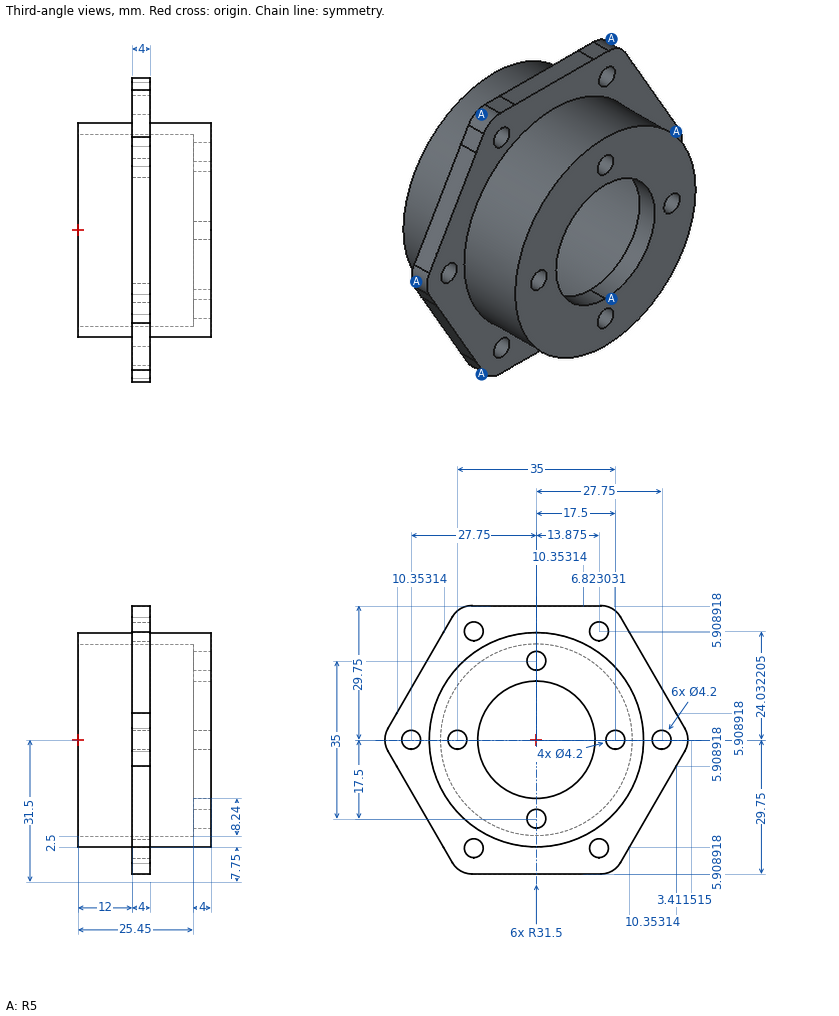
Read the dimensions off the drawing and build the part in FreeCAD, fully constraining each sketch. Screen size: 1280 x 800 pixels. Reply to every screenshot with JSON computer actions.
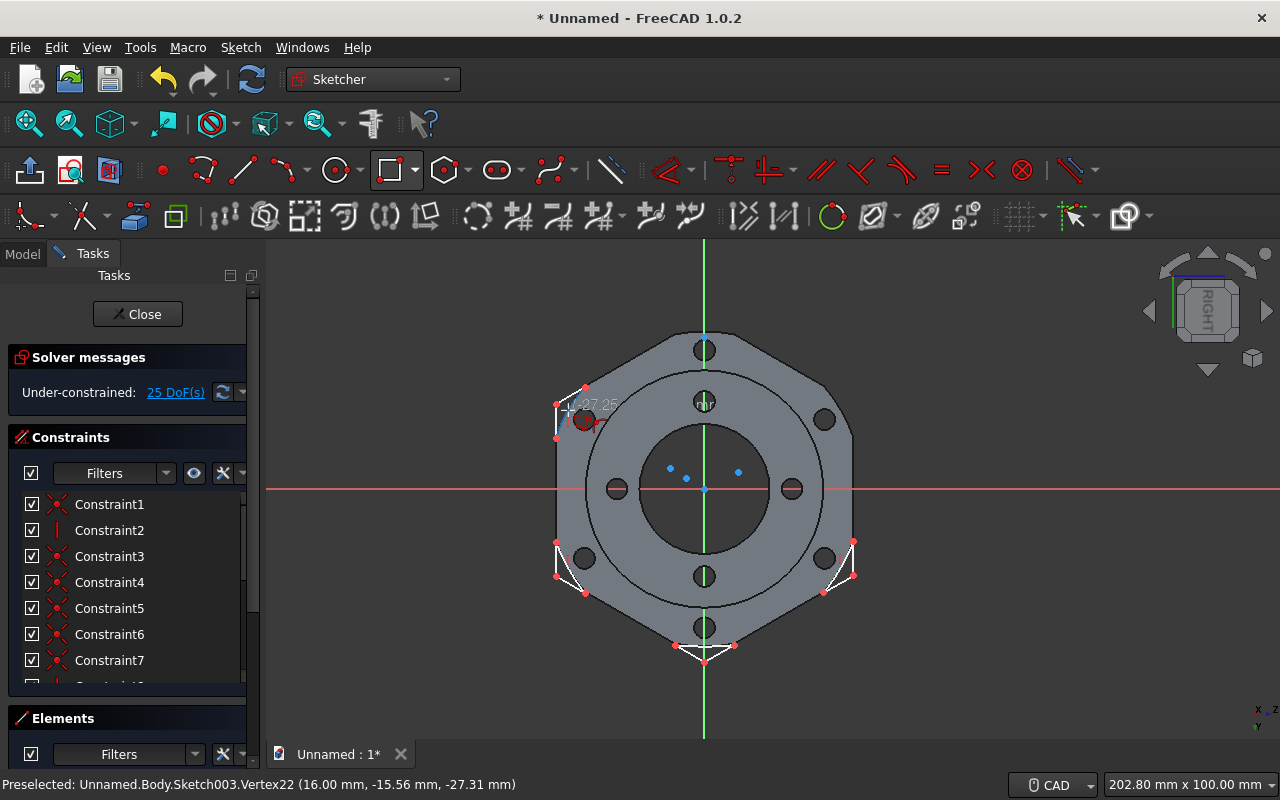
{"action": "left_click", "coordinate": [734, 334]}
{"action": "left_click", "coordinate": [704, 317]}
{"action": "left_click", "coordinate": [675, 334]}
{"action": "right_click", "coordinate": [675, 334]}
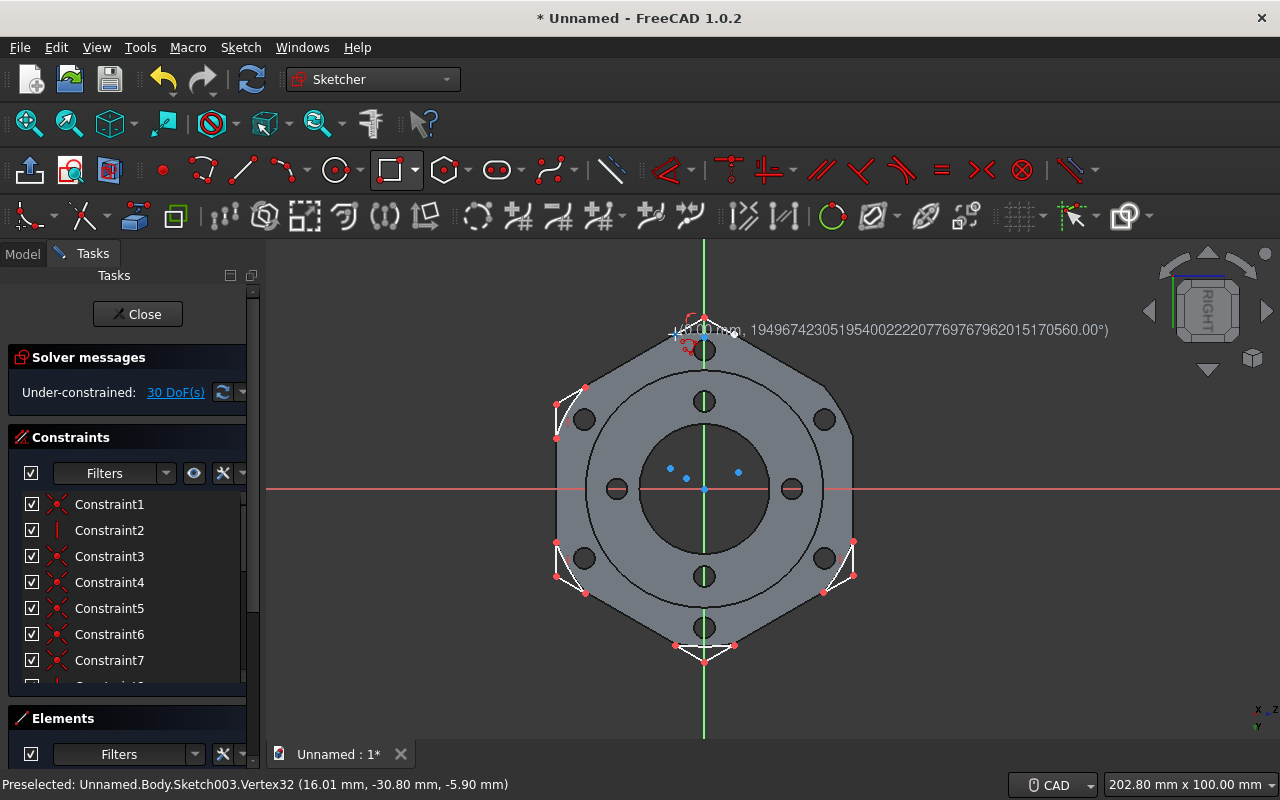
{"action": "key", "text": "g 3 a"}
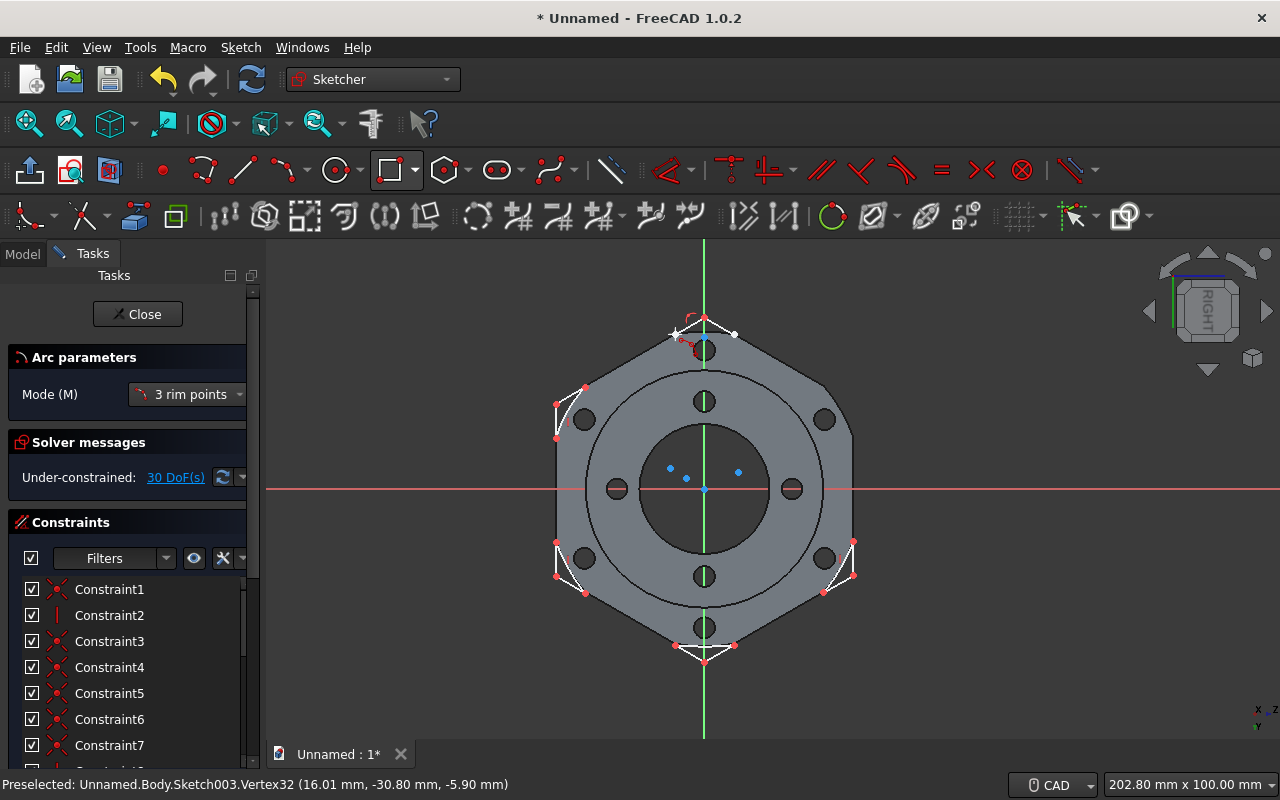
{"action": "left_click", "coordinate": [675, 335]}
{"action": "left_click", "coordinate": [734, 335]}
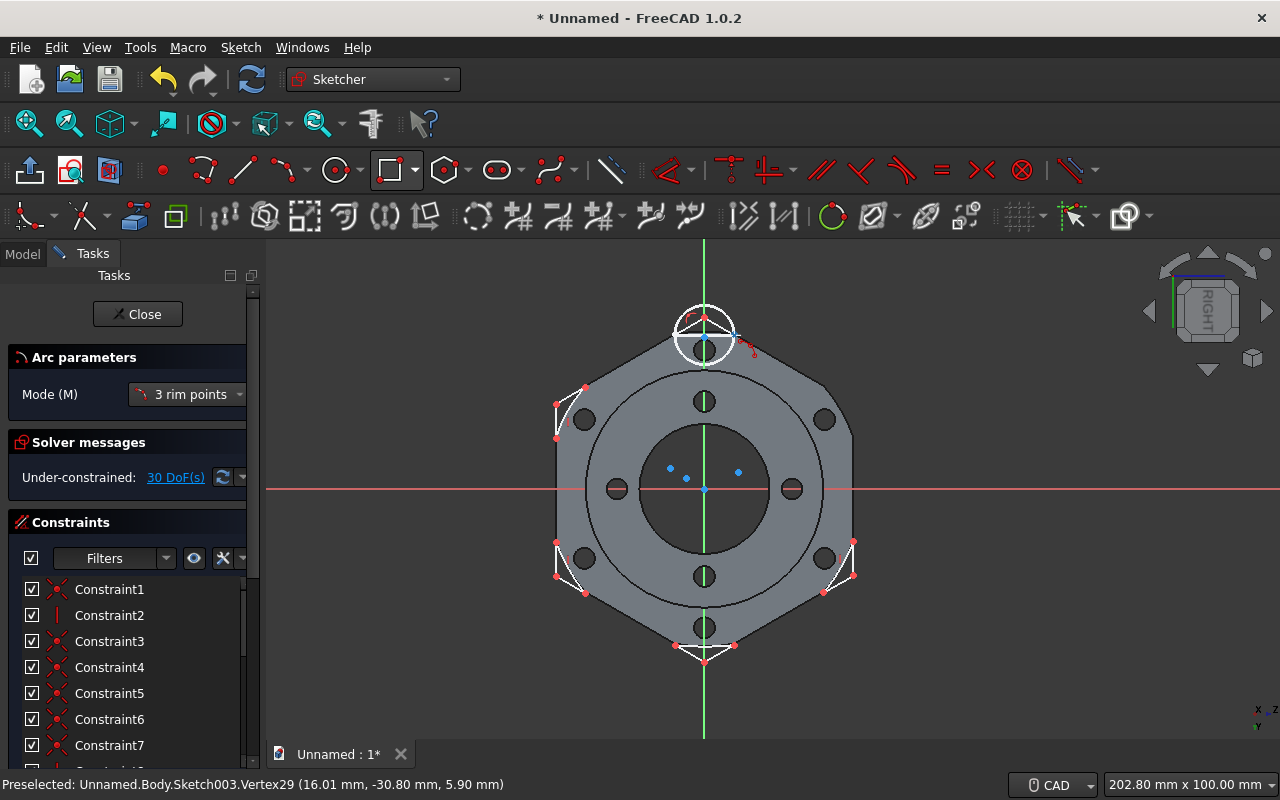
{"action": "scroll", "coordinate": [710, 332], "scroll_direction": "up", "scroll_amount": 9}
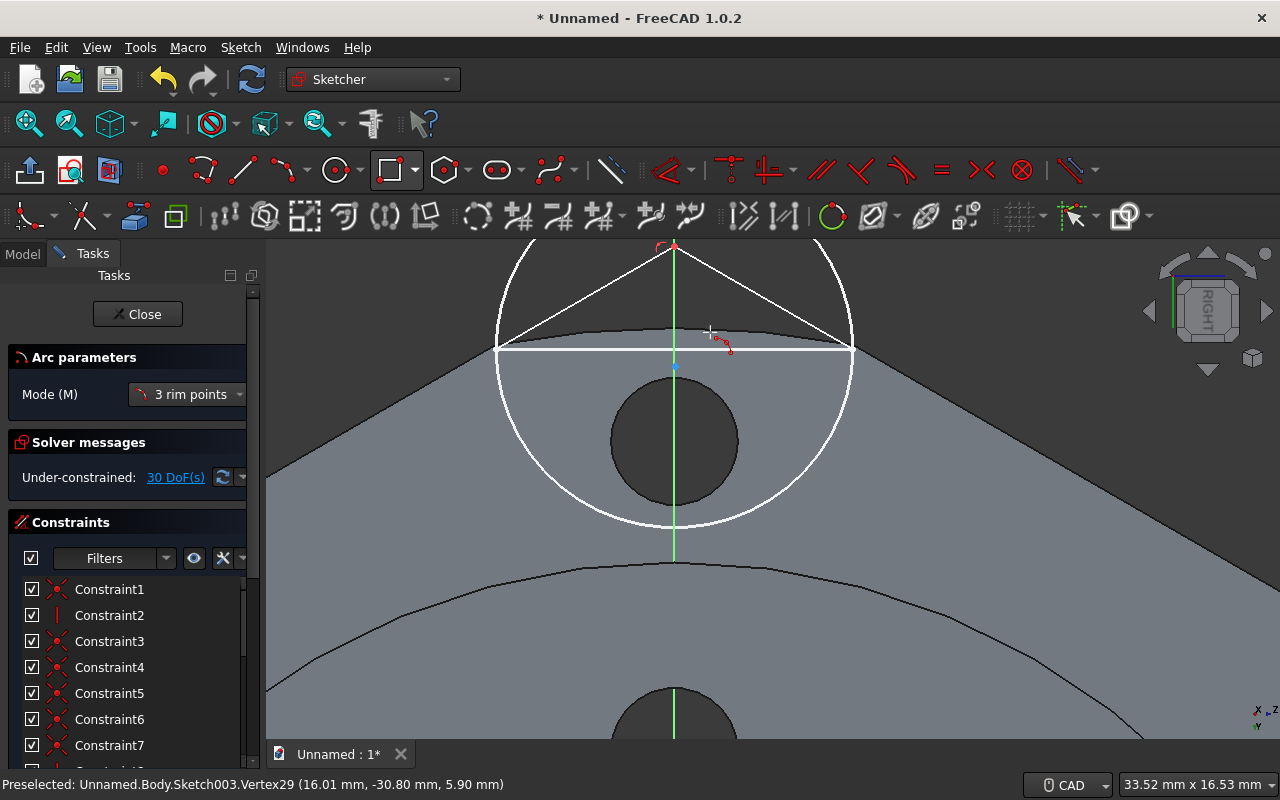
{"action": "left_click", "coordinate": [710, 329]}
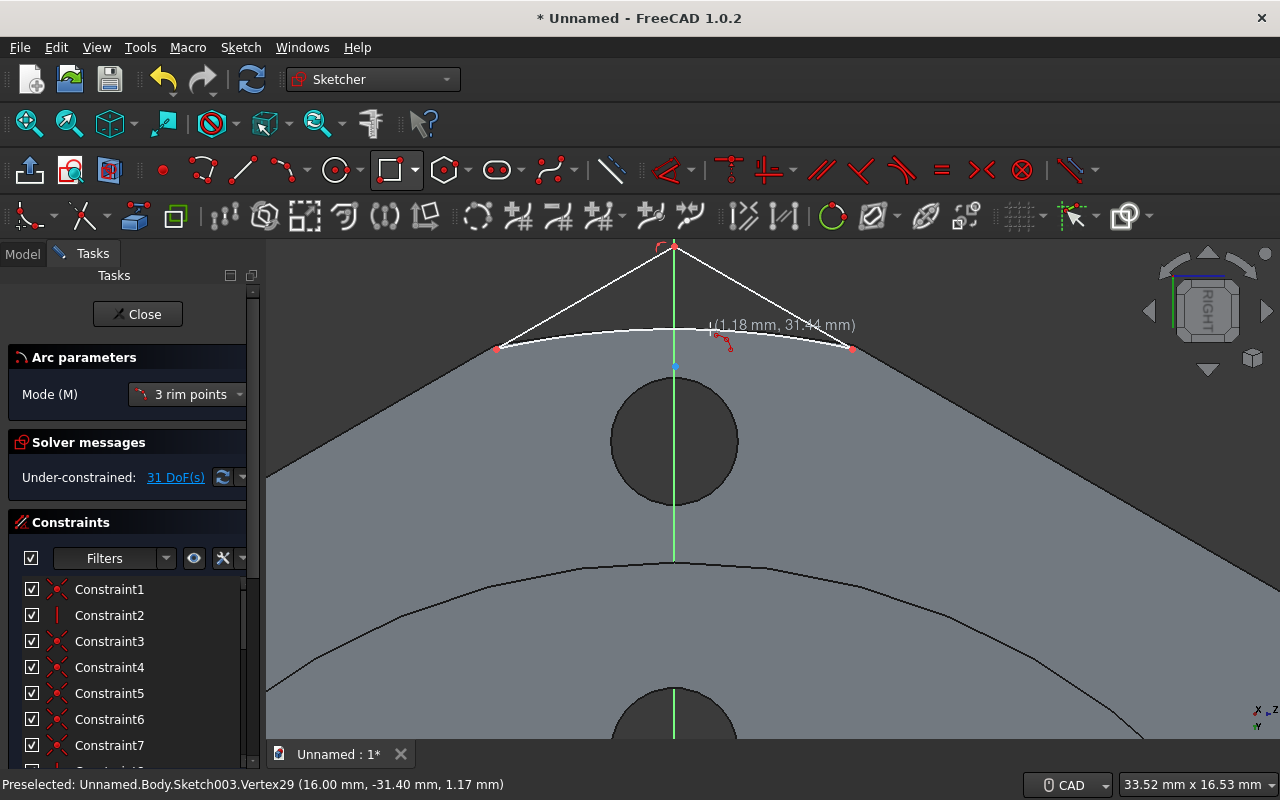
{"action": "key", "text": "g m"}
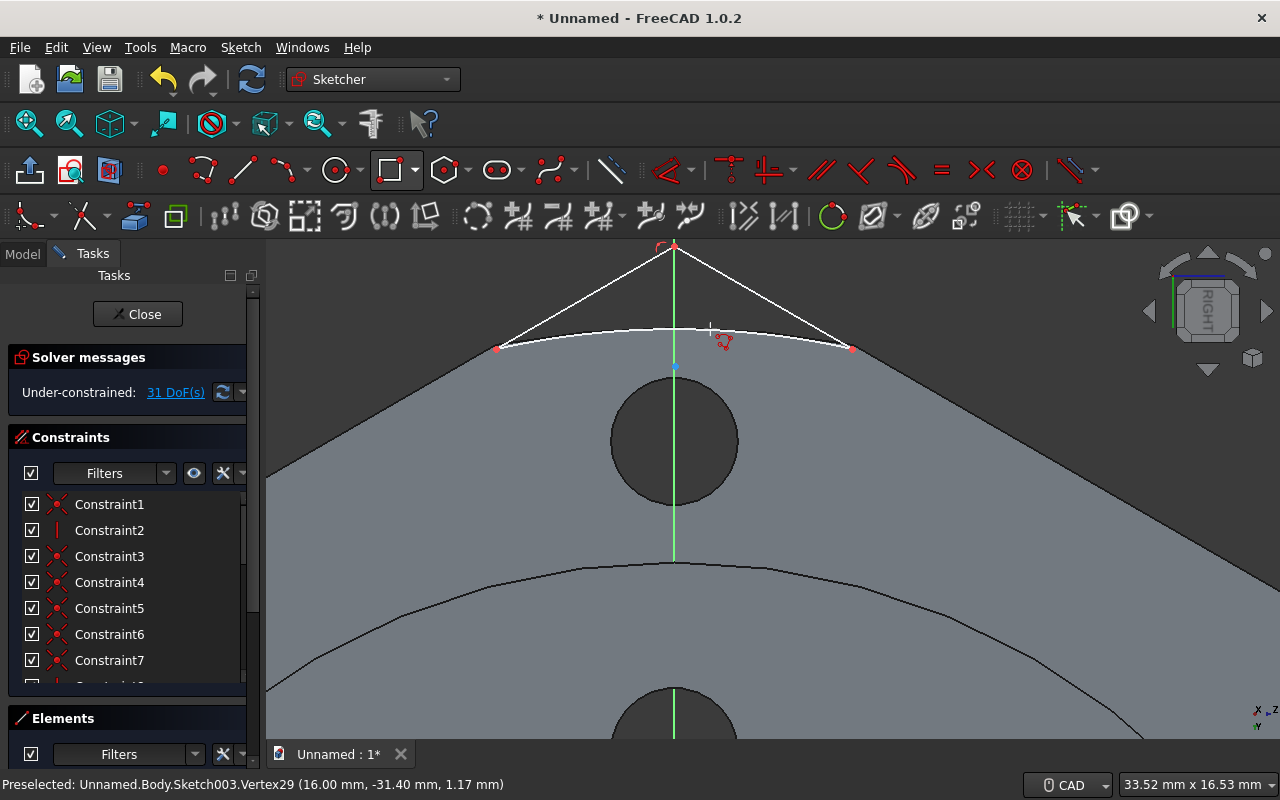
{"action": "scroll", "coordinate": [710, 332], "scroll_direction": "down", "scroll_amount": 9}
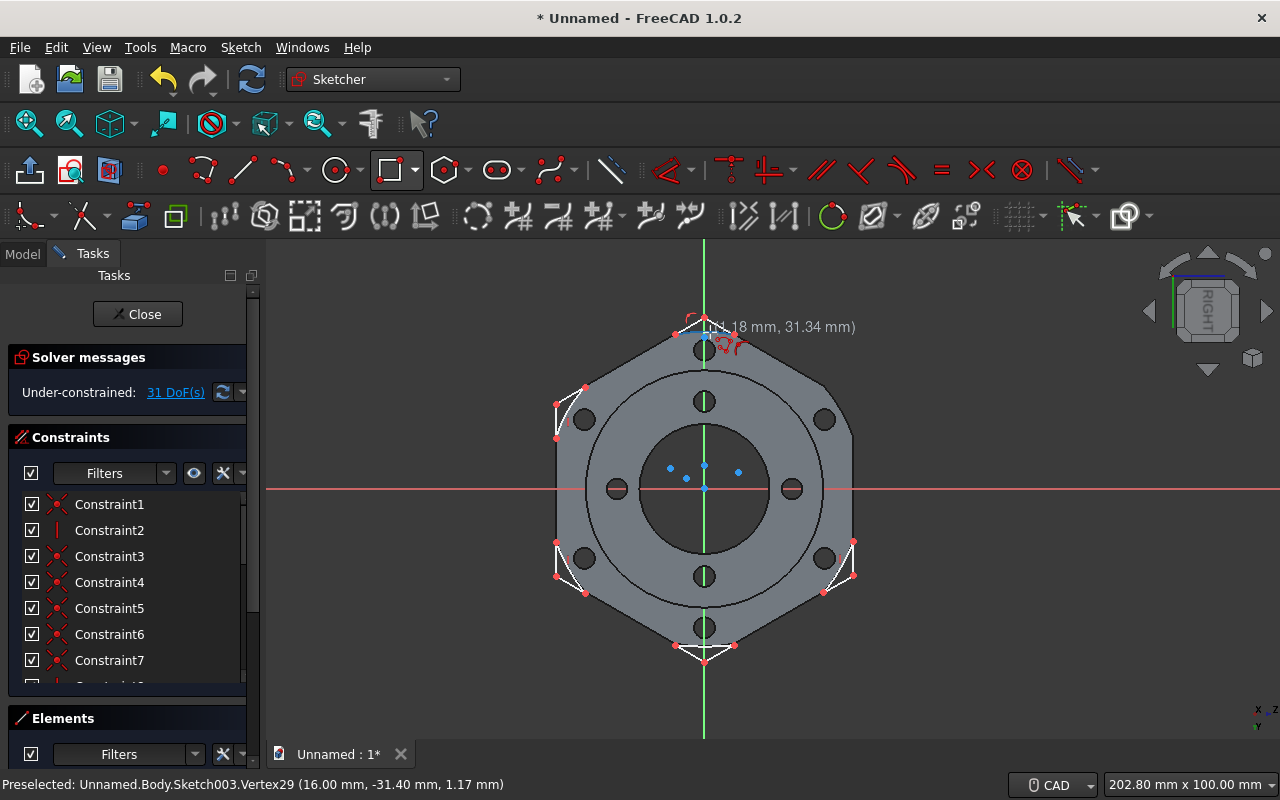
{"action": "left_click", "coordinate": [853, 437]}
{"action": "left_click", "coordinate": [853, 403]}
{"action": "left_click", "coordinate": [824, 386]}
{"action": "right_click", "coordinate": [824, 386]}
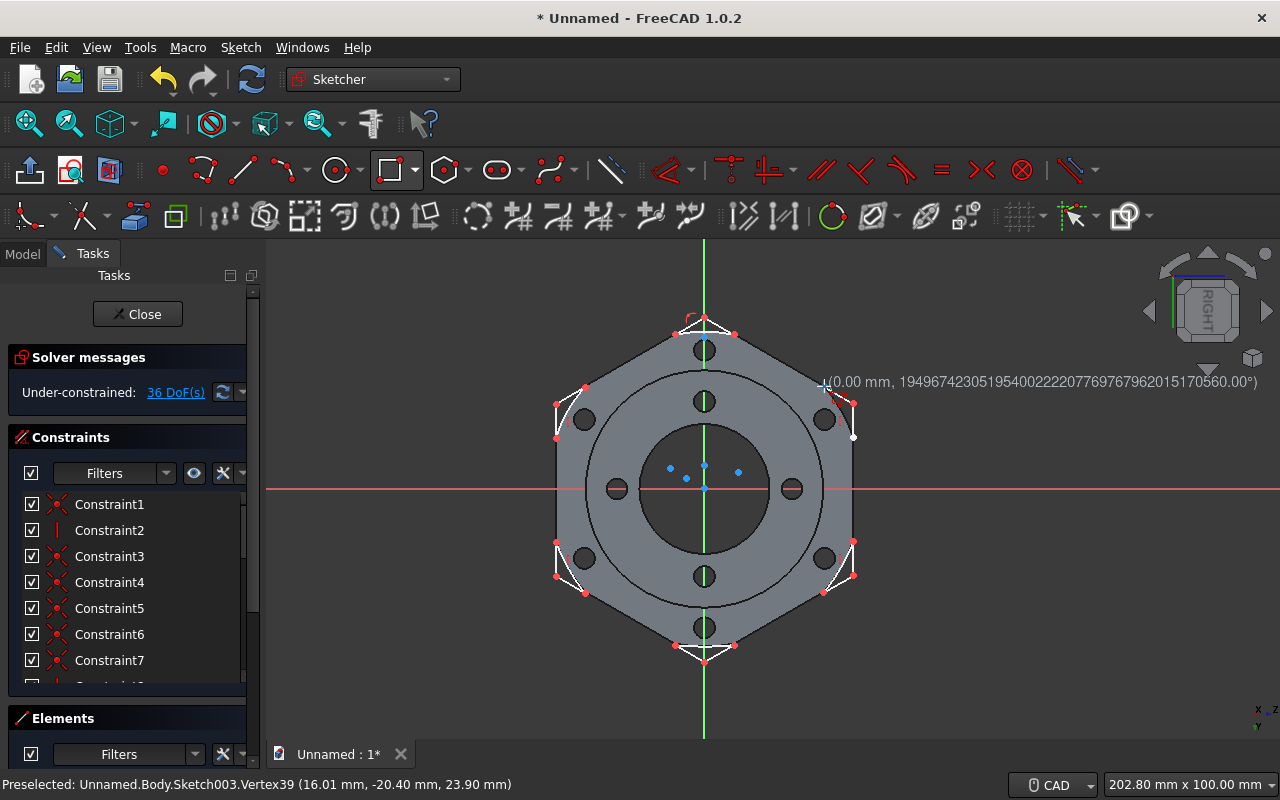
{"action": "key", "text": "g 3 a"}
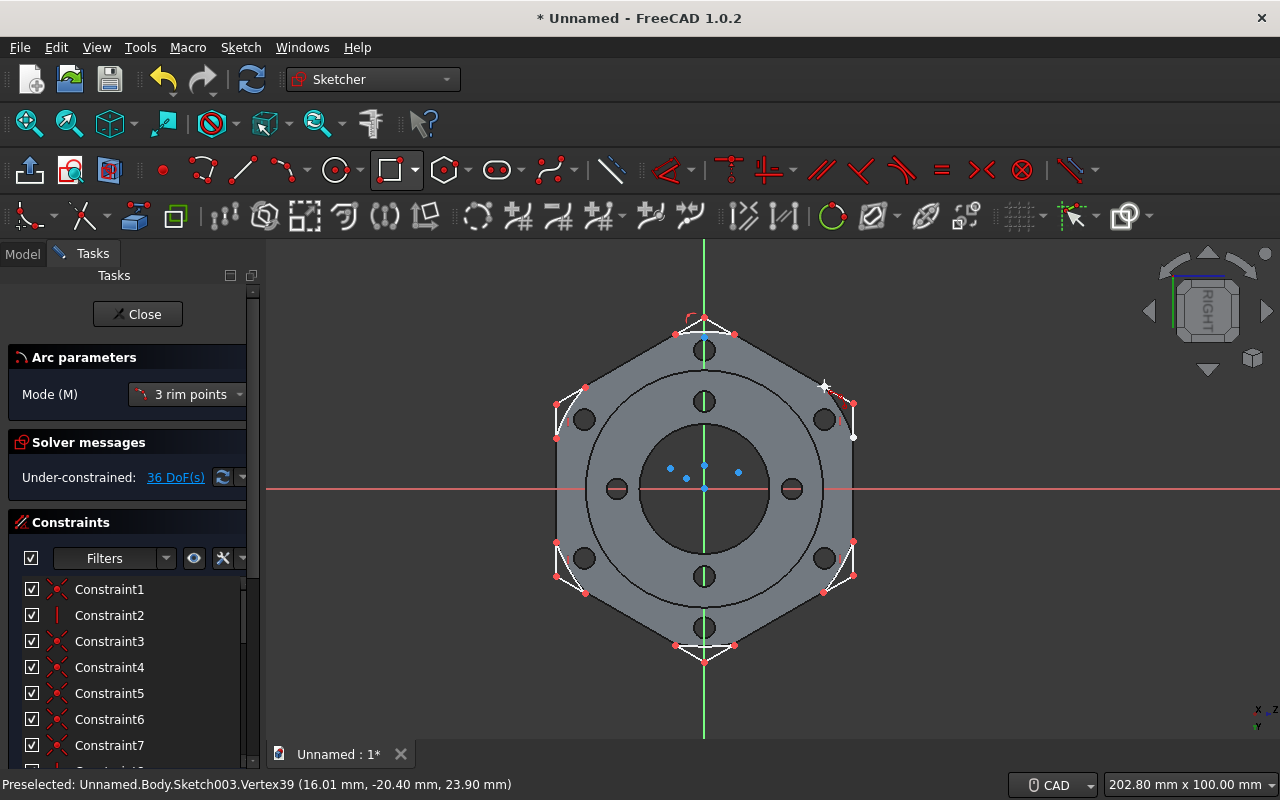
{"action": "left_click", "coordinate": [824, 387]}
{"action": "left_click", "coordinate": [853, 438]}